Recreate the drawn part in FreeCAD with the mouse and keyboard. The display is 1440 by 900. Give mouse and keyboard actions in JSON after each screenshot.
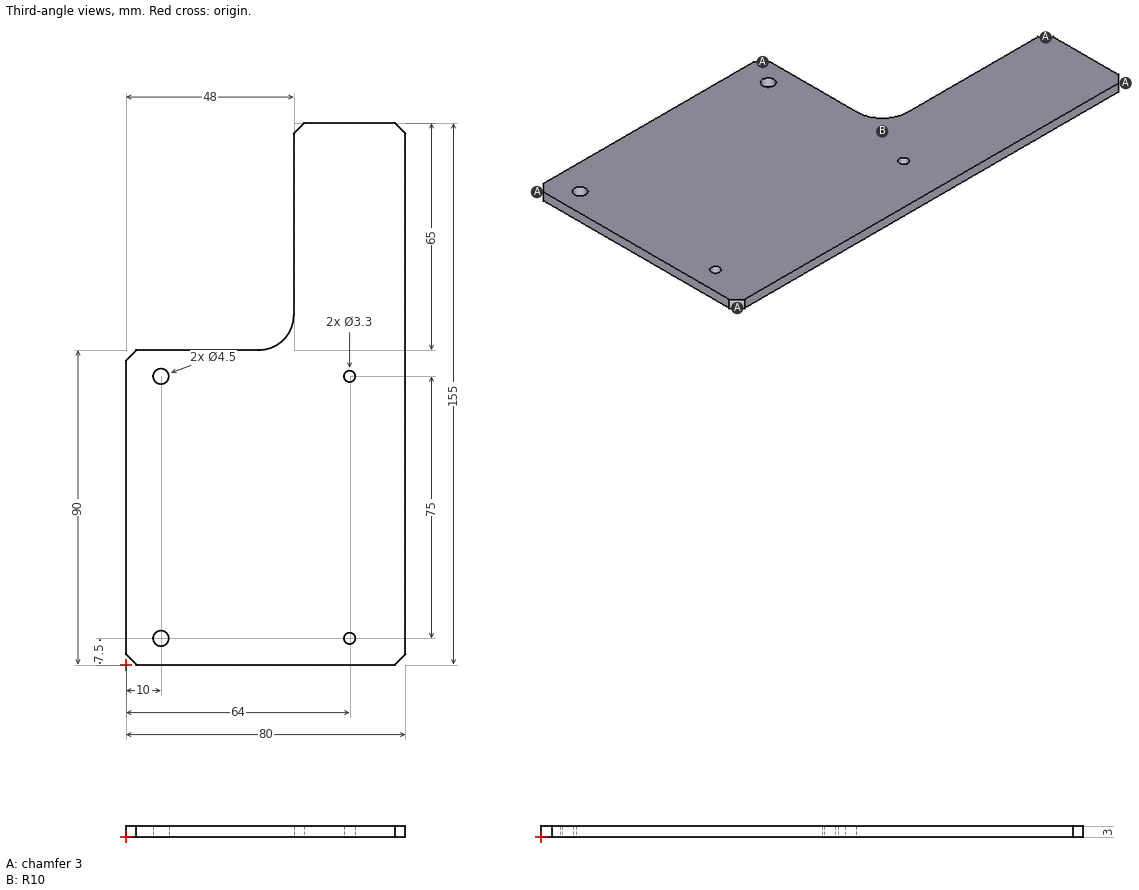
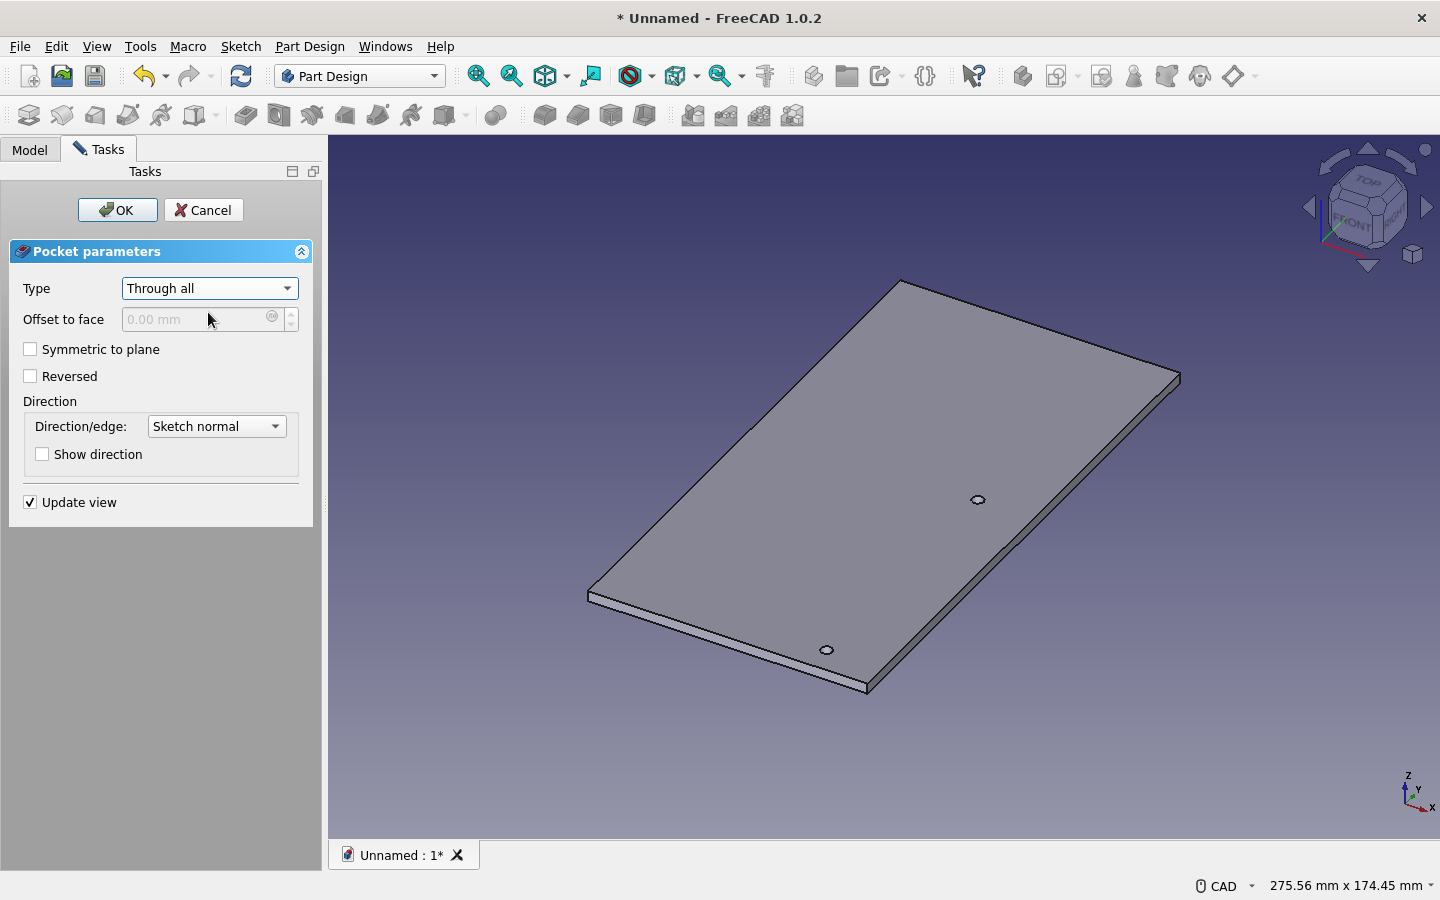
{"action": "left_click", "coordinate": [118, 210]}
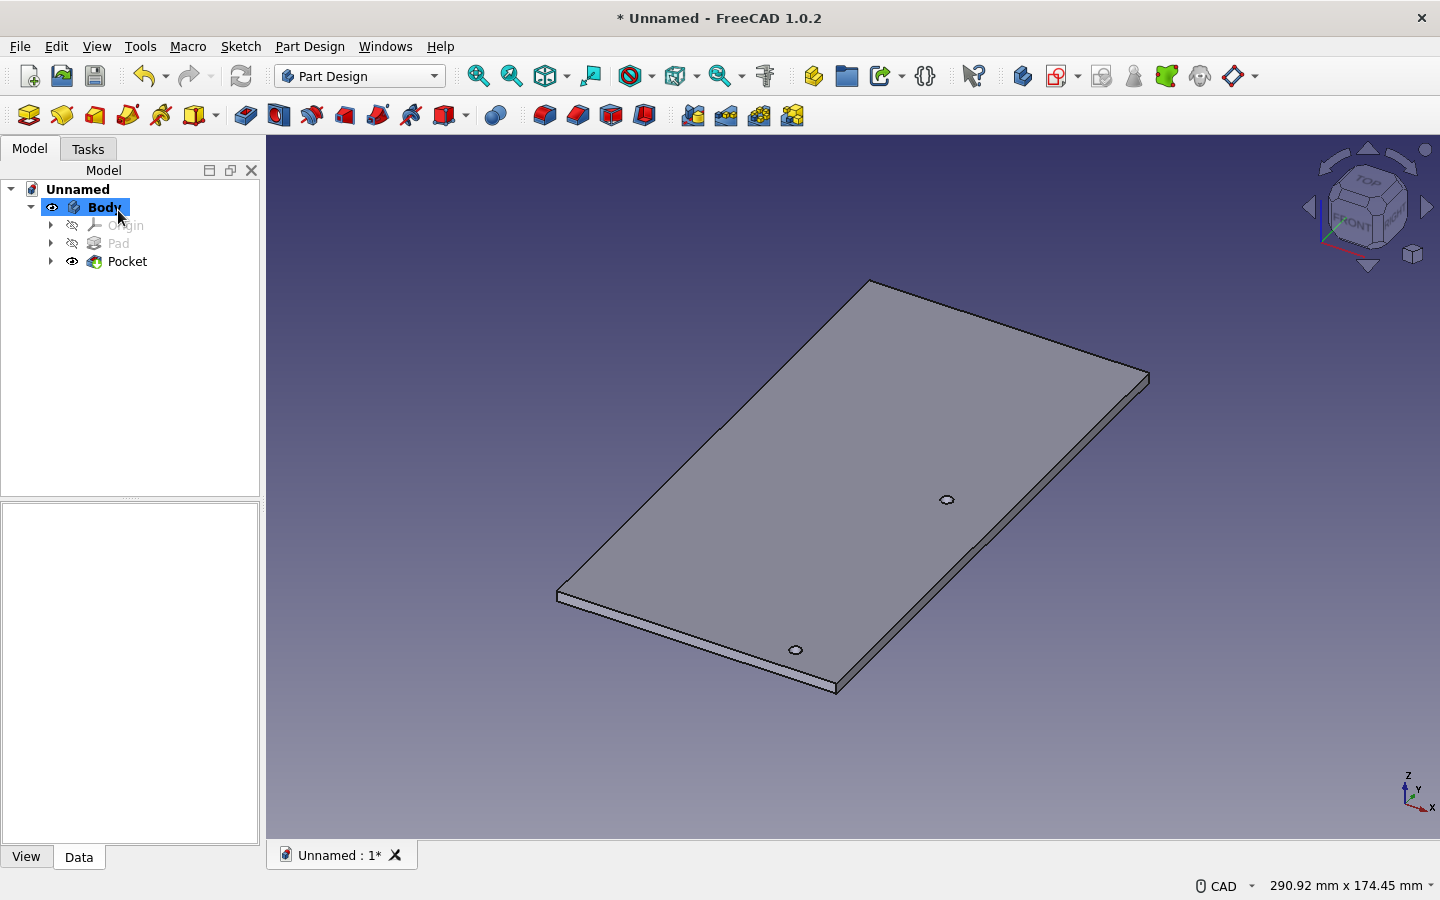
{"action": "left_click", "coordinate": [808, 525]}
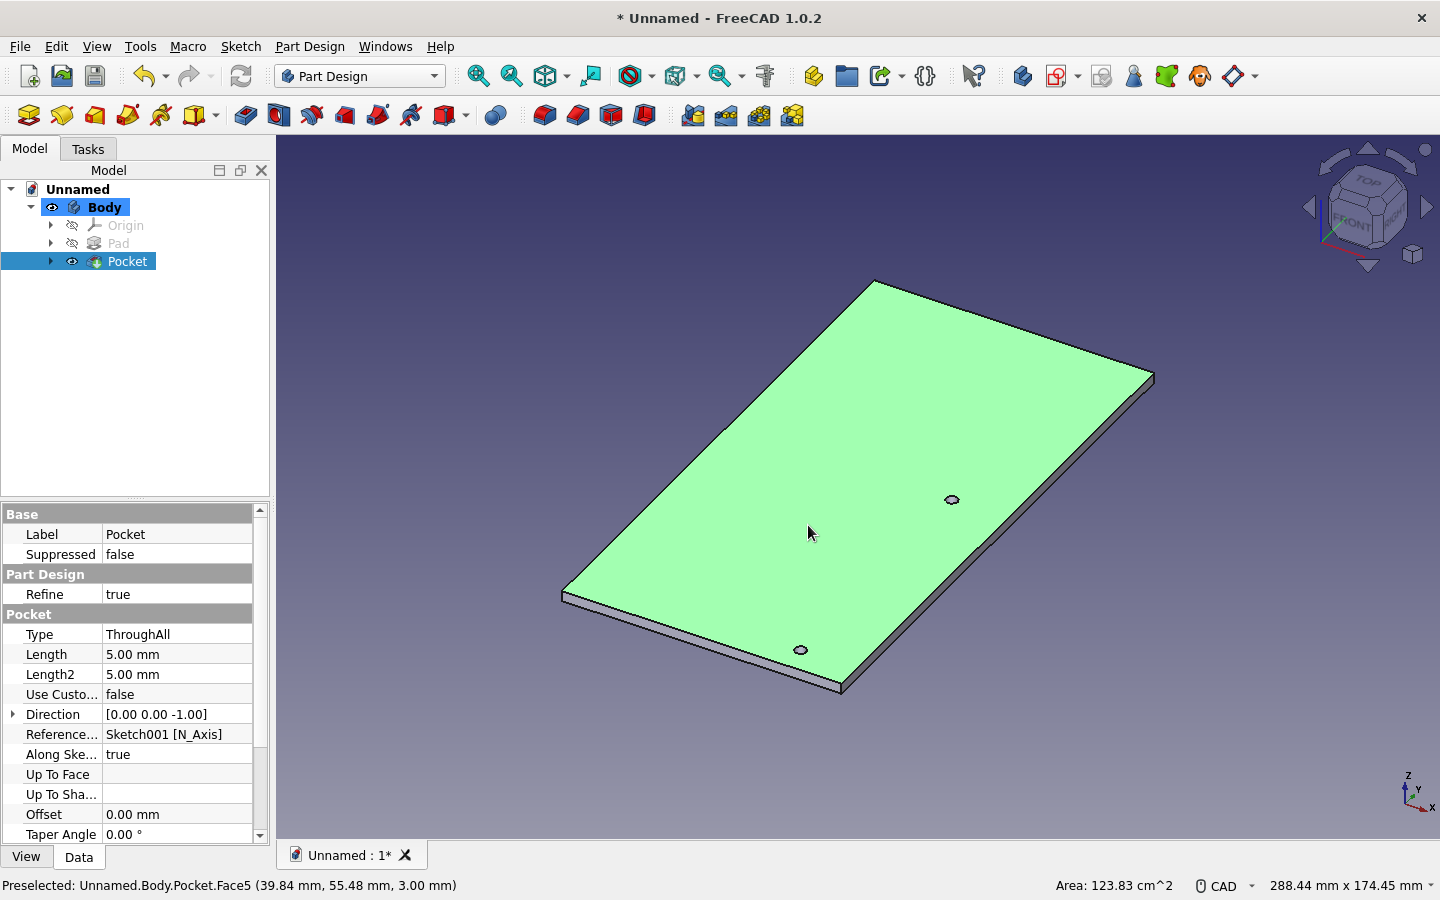
{"action": "left_click", "coordinate": [1056, 76]}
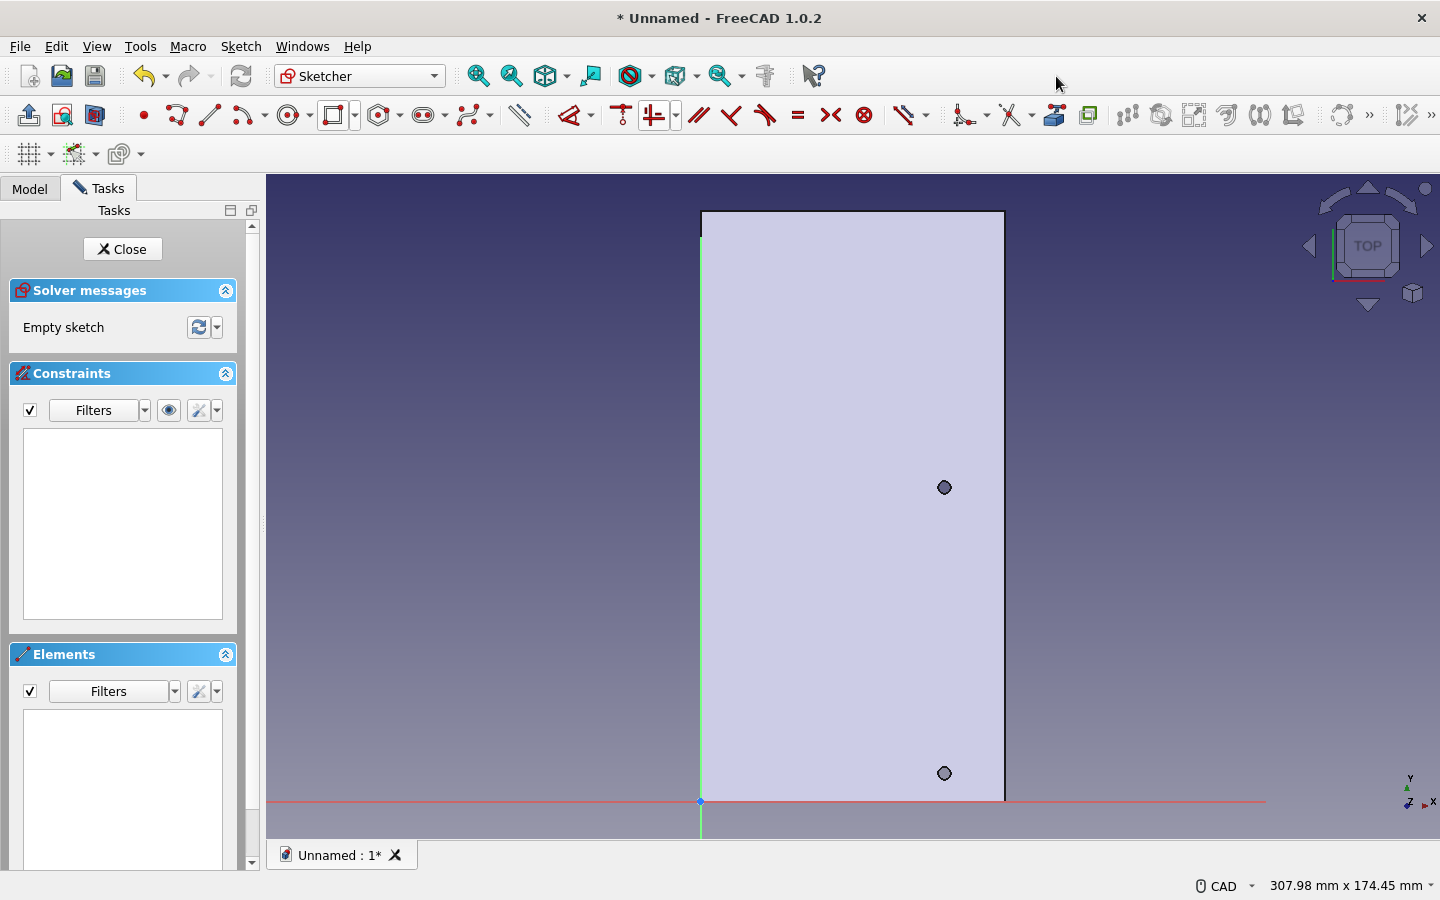
{"action": "scroll", "coordinate": [1058, 202], "scroll_direction": "down", "scroll_amount": 1}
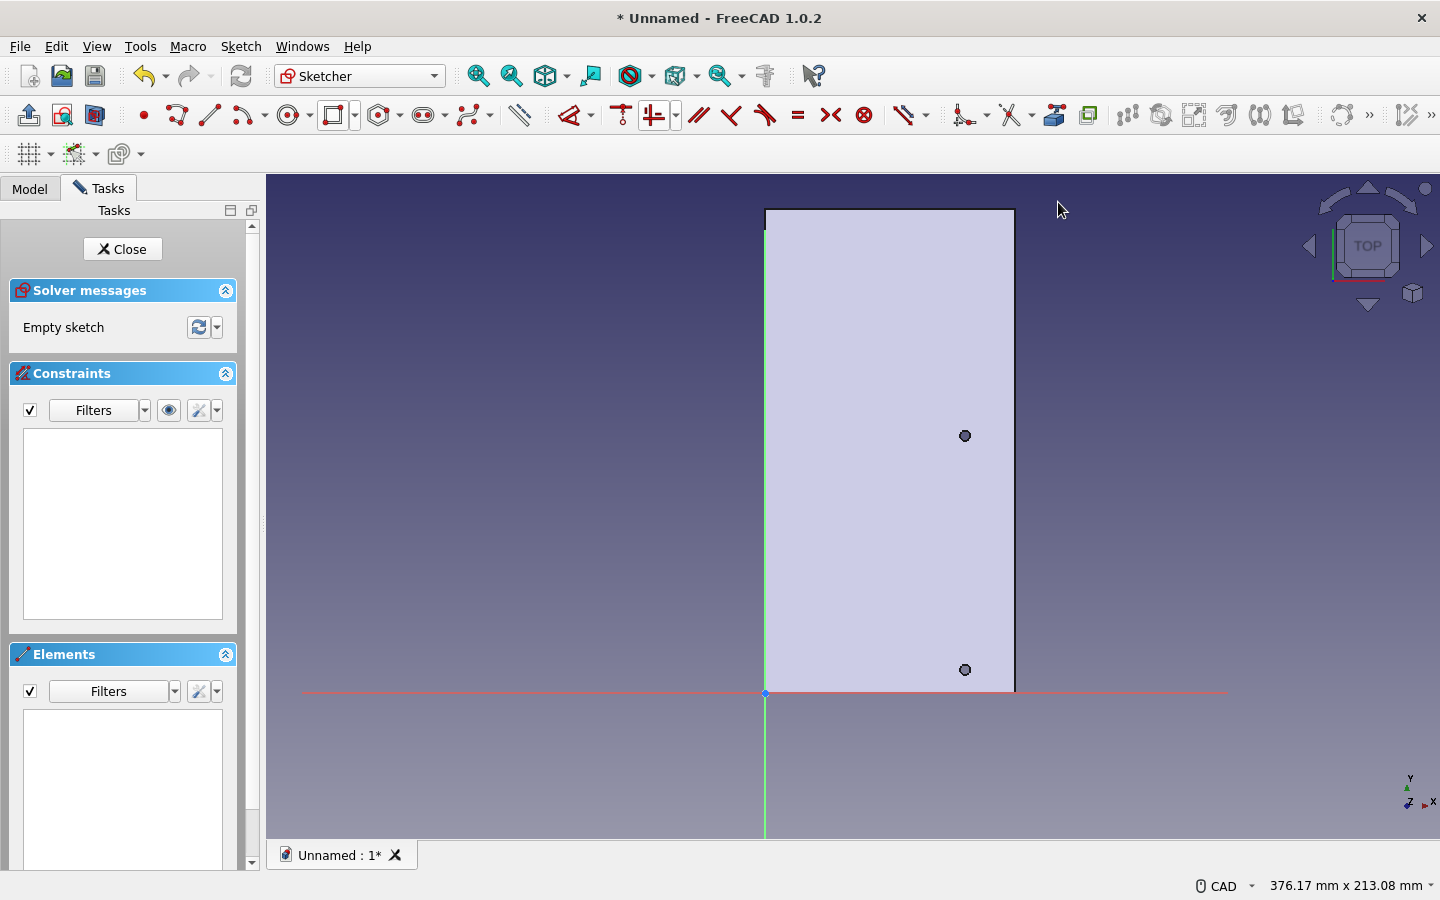
{"action": "scroll", "coordinate": [785, 672], "scroll_direction": "up", "scroll_amount": 2}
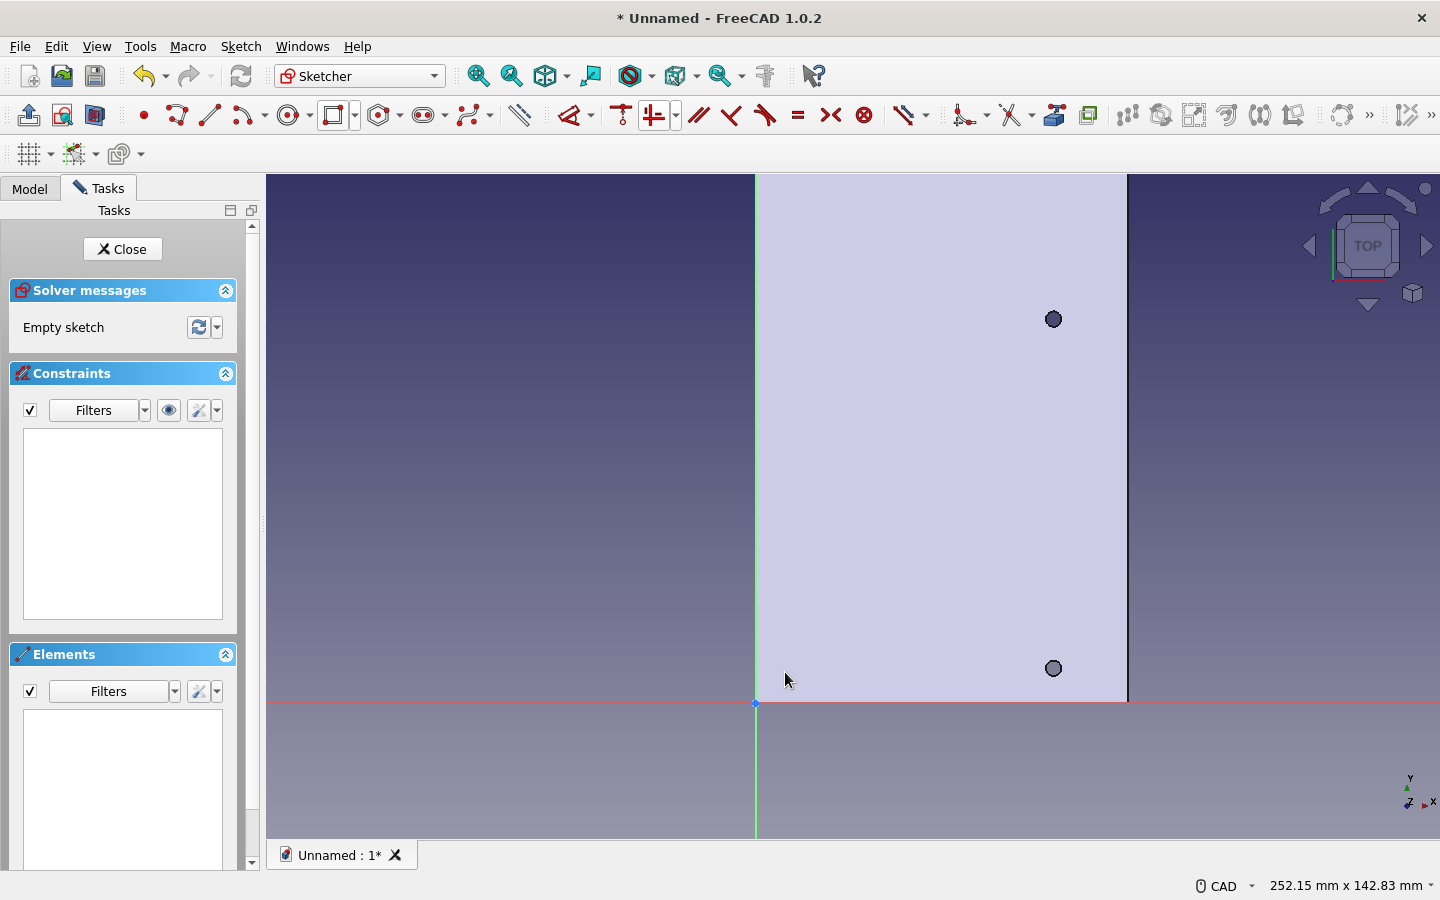
{"action": "left_click", "coordinate": [288, 116]}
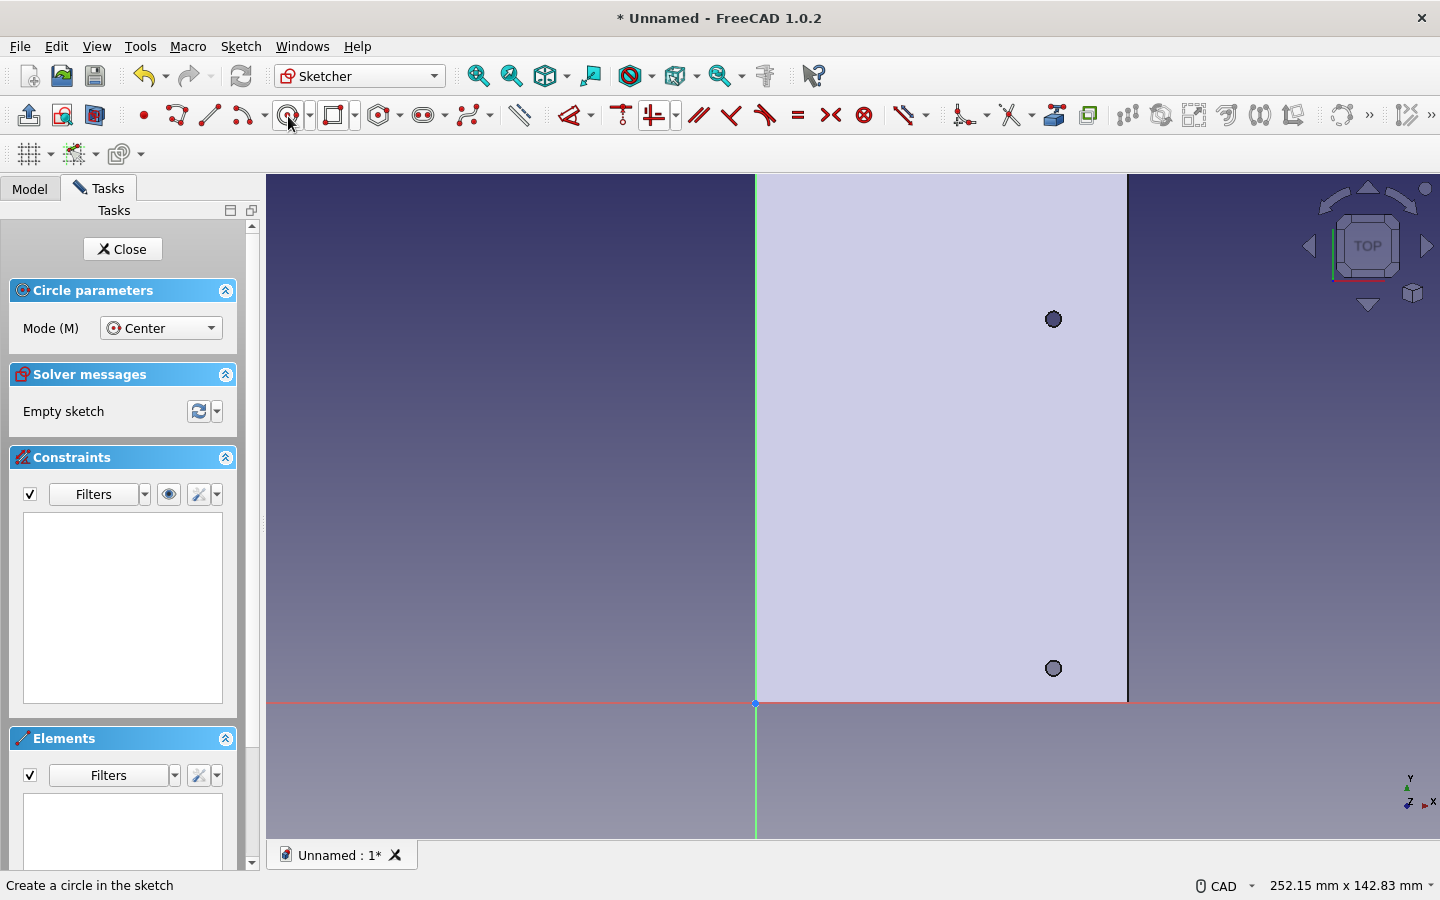
{"action": "scroll", "coordinate": [802, 319], "scroll_direction": "up", "scroll_amount": 4}